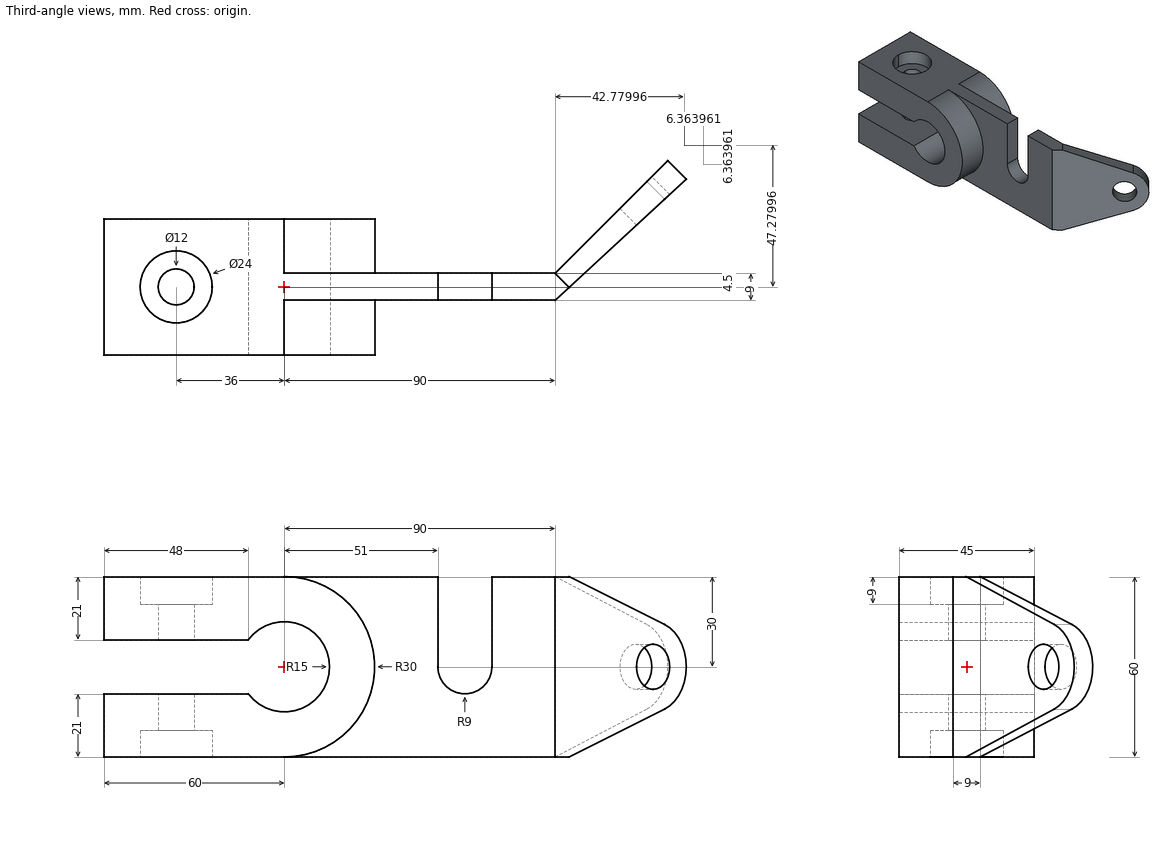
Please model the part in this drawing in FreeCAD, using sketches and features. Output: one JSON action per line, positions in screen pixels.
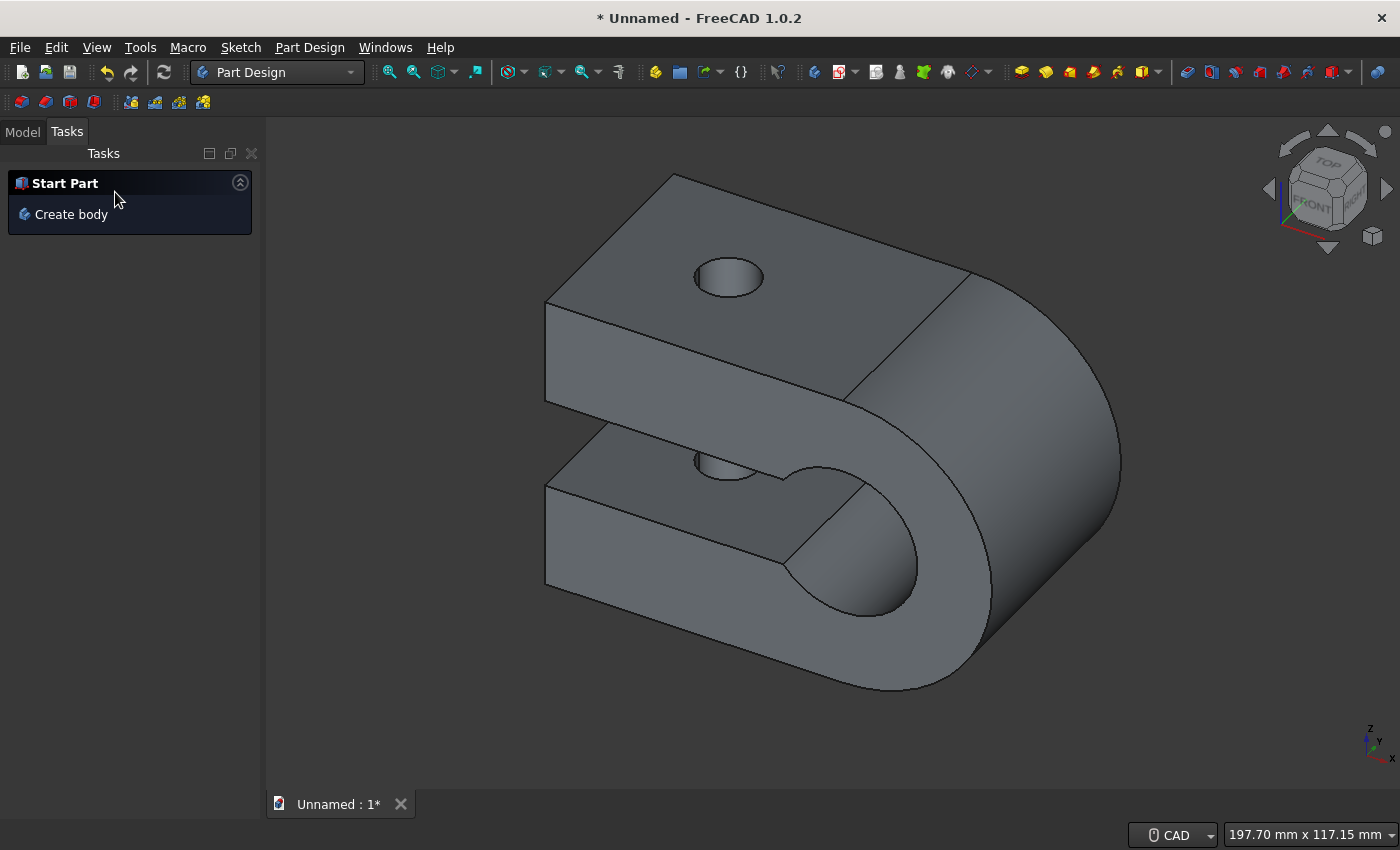
{"action": "left_click", "coordinate": [862, 296]}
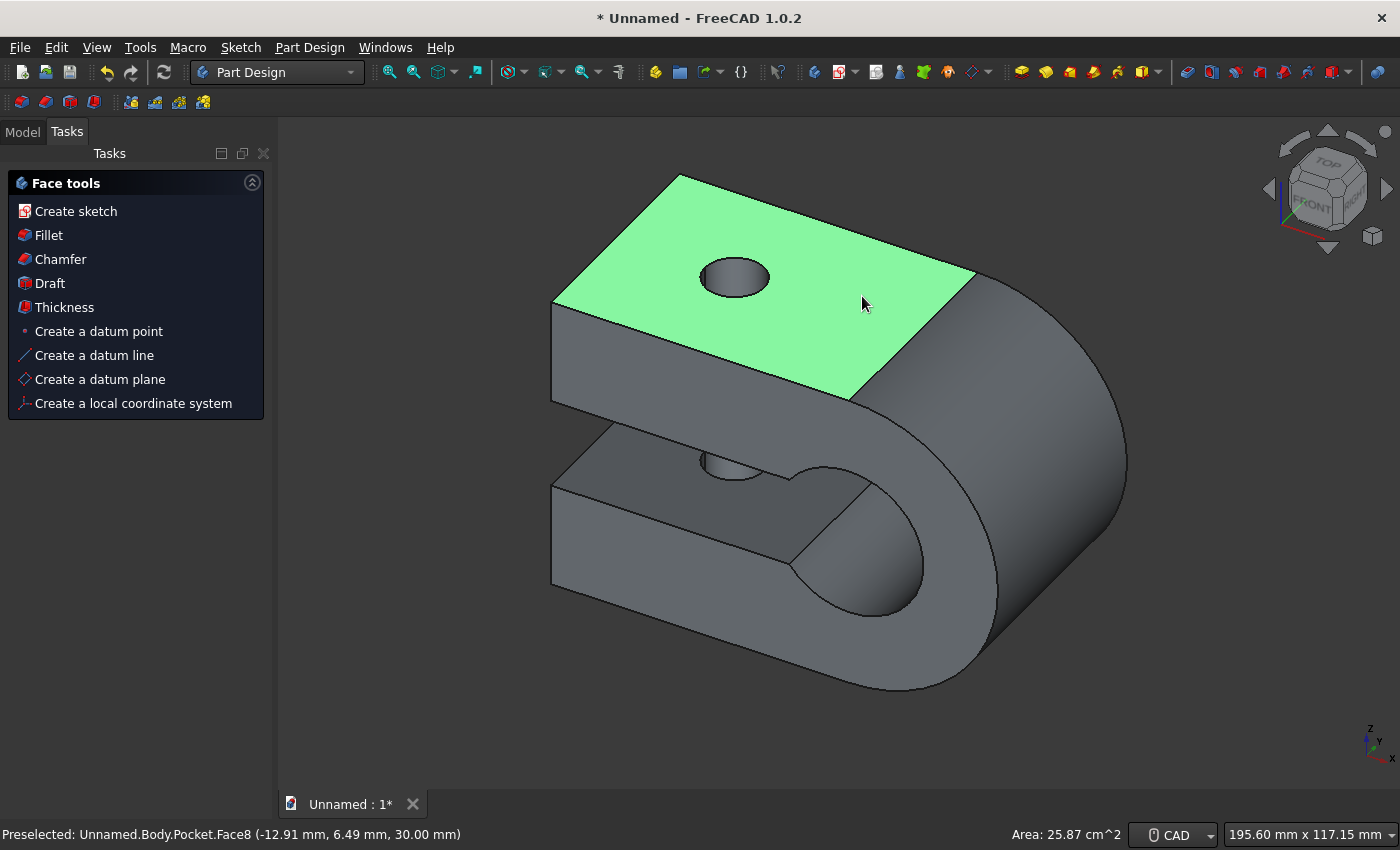
{"action": "left_click", "coordinate": [840, 72]}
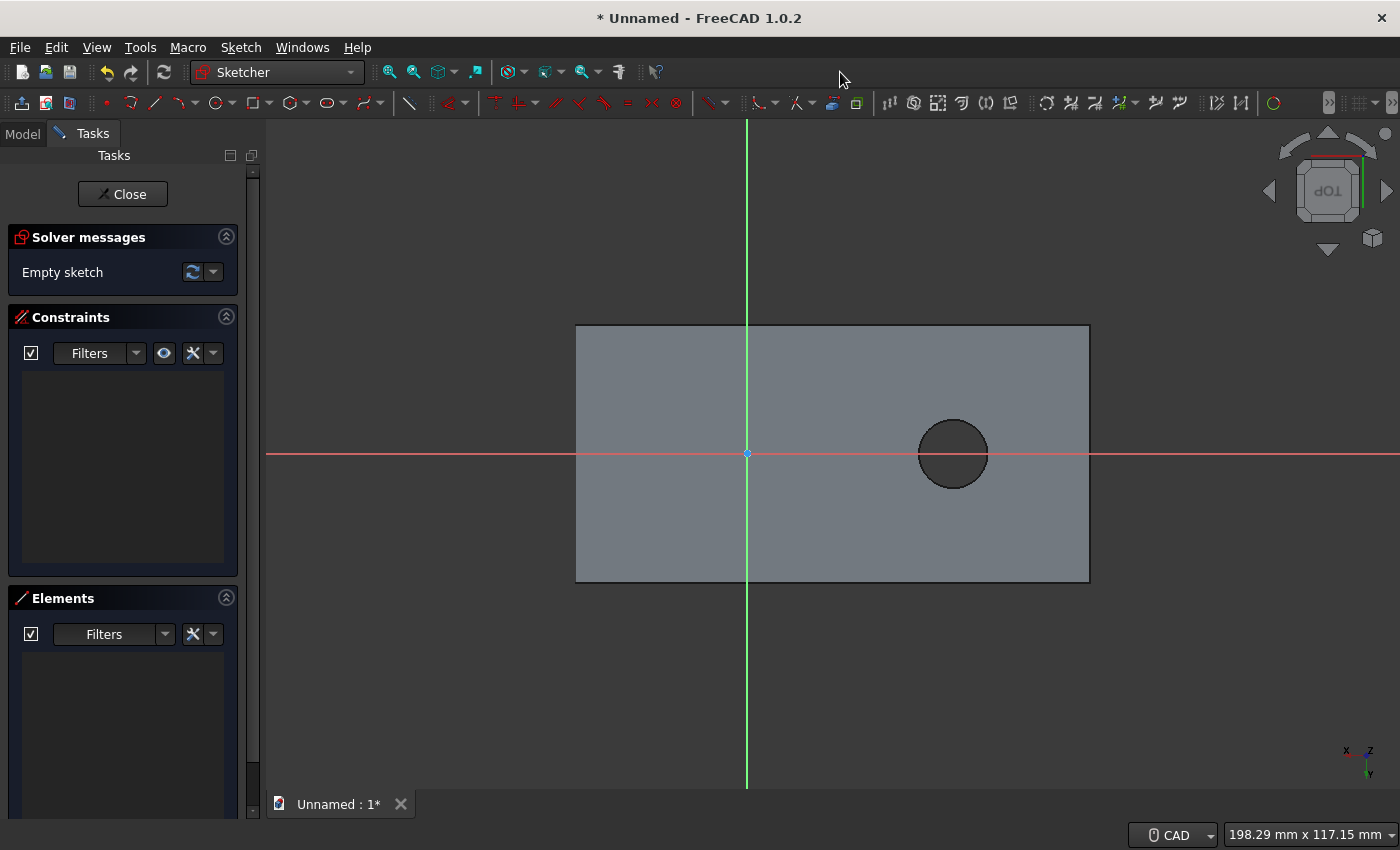
{"action": "scroll", "coordinate": [982, 454], "scroll_direction": "up", "scroll_amount": 4}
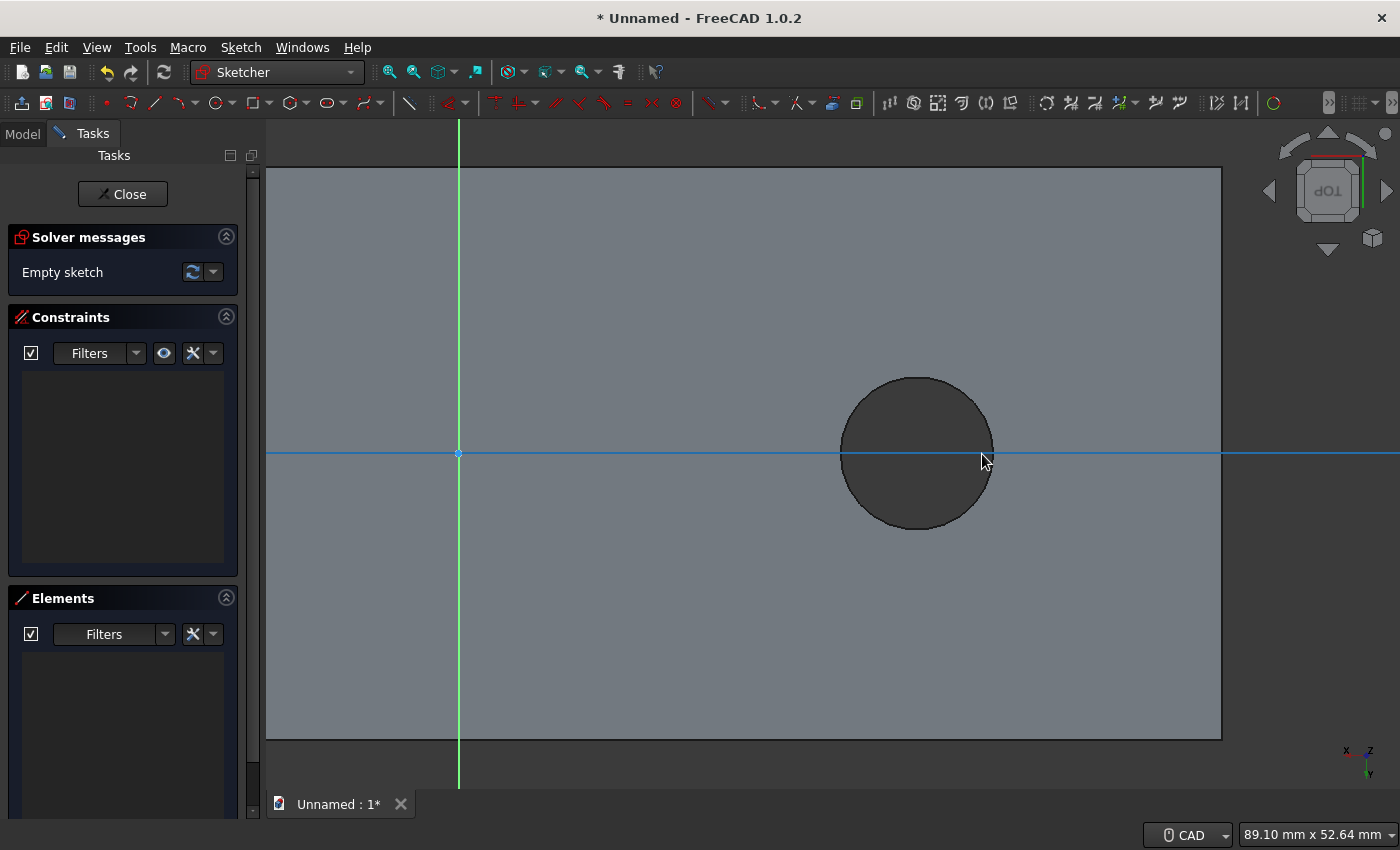
{"action": "key", "text": "g c"}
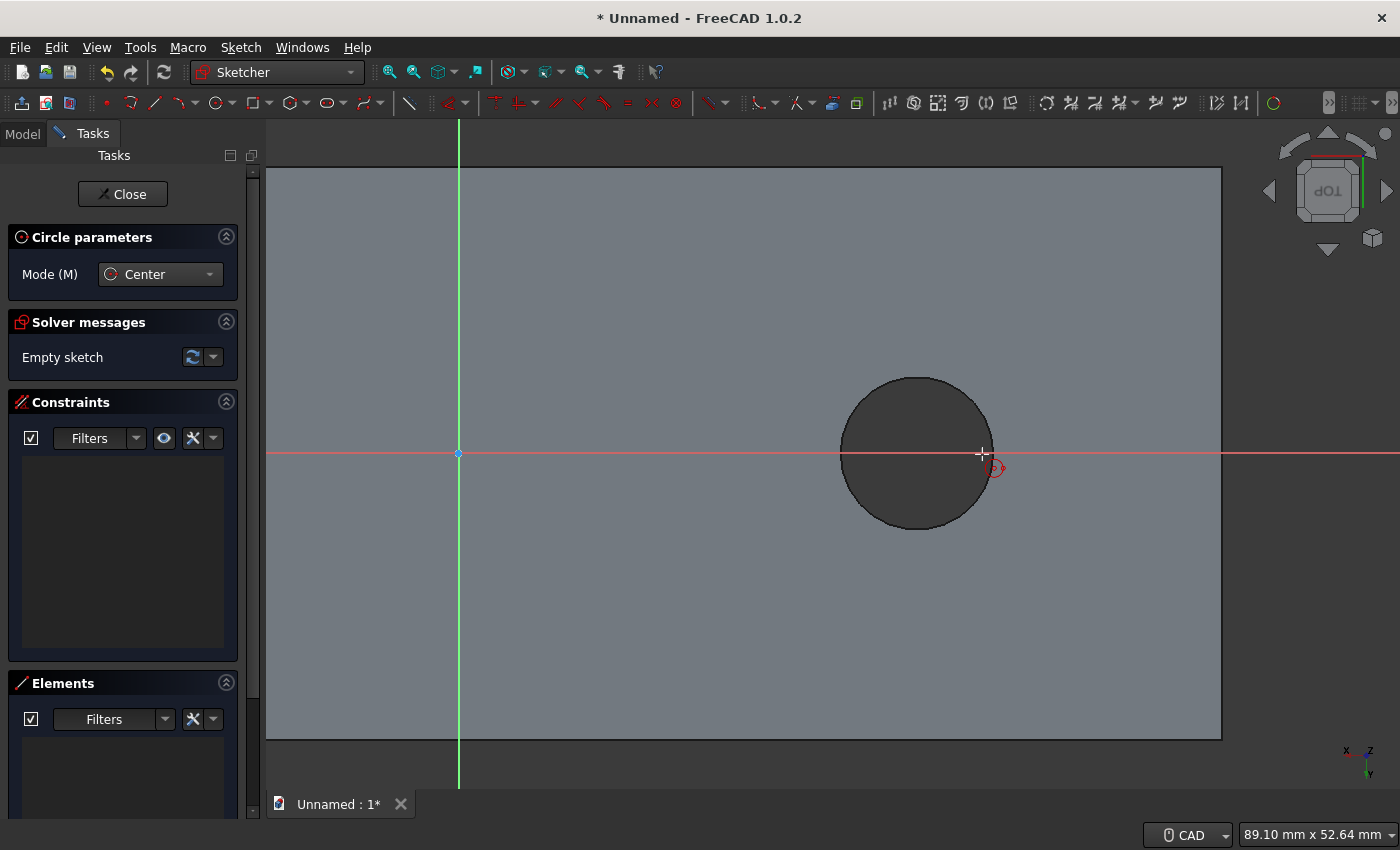
{"action": "left_click", "coordinate": [917, 453]}
{"action": "left_click", "coordinate": [1025, 345]}
{"action": "key", "text": "Escape"}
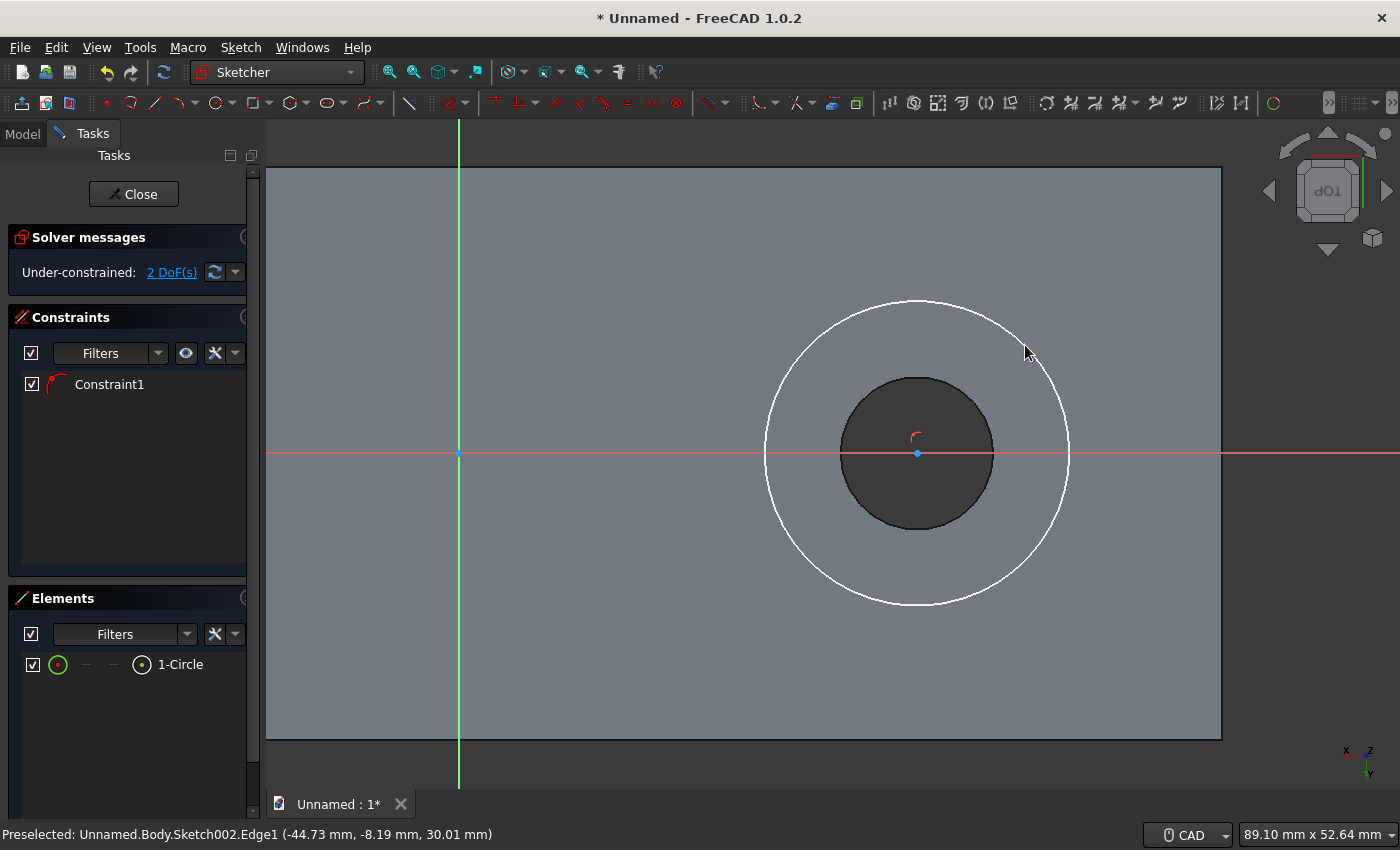
{"action": "key", "text": "d"}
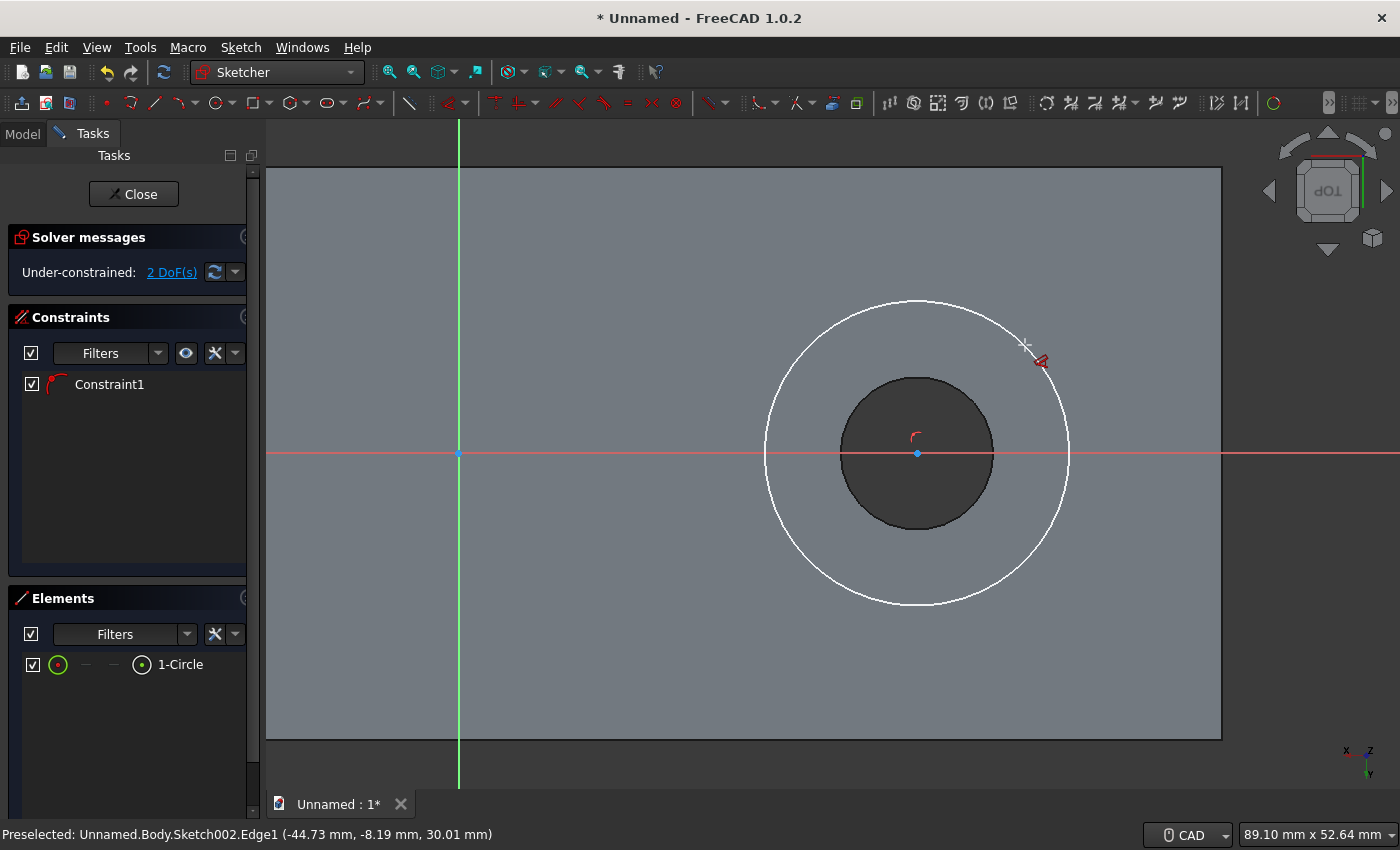
{"action": "left_click", "coordinate": [1024, 345]}
{"action": "left_click", "coordinate": [1046, 322]}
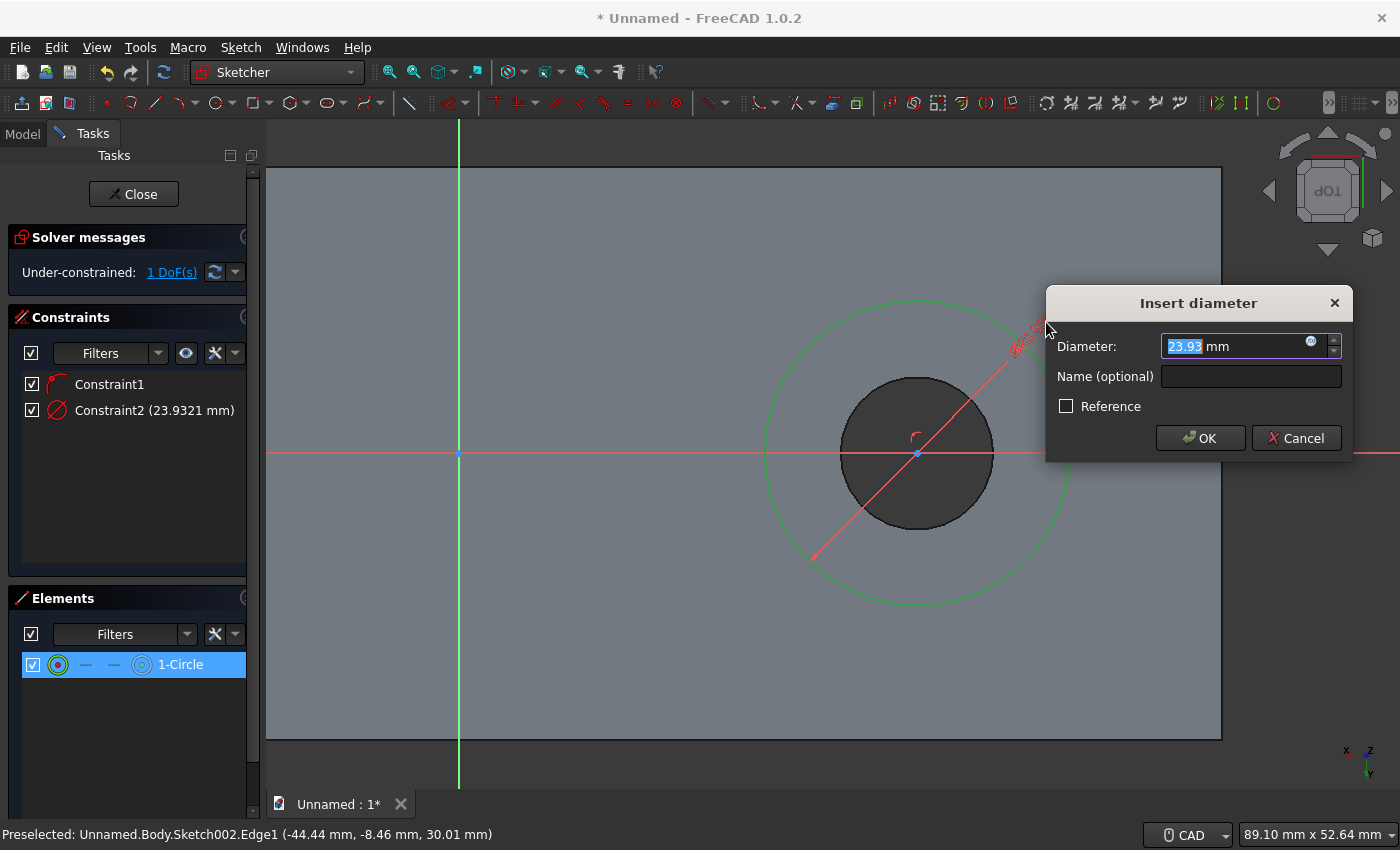
{"action": "type", "text": "24"}
{"action": "key", "text": "Return"}